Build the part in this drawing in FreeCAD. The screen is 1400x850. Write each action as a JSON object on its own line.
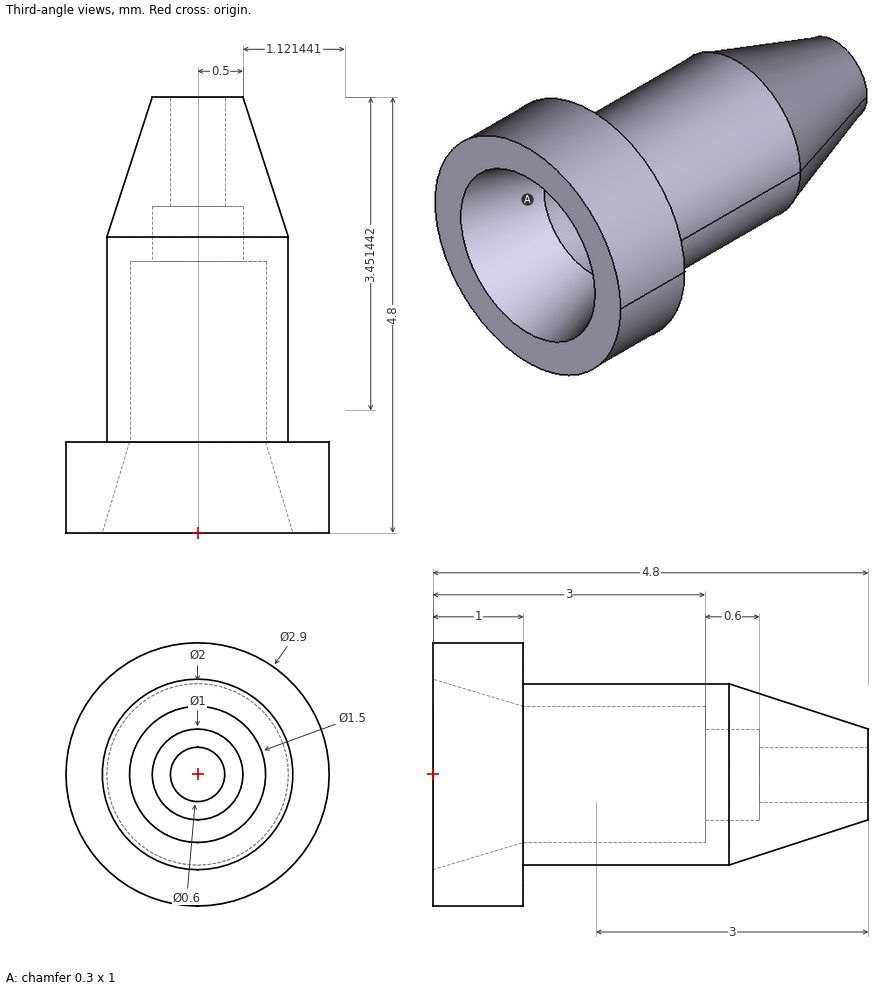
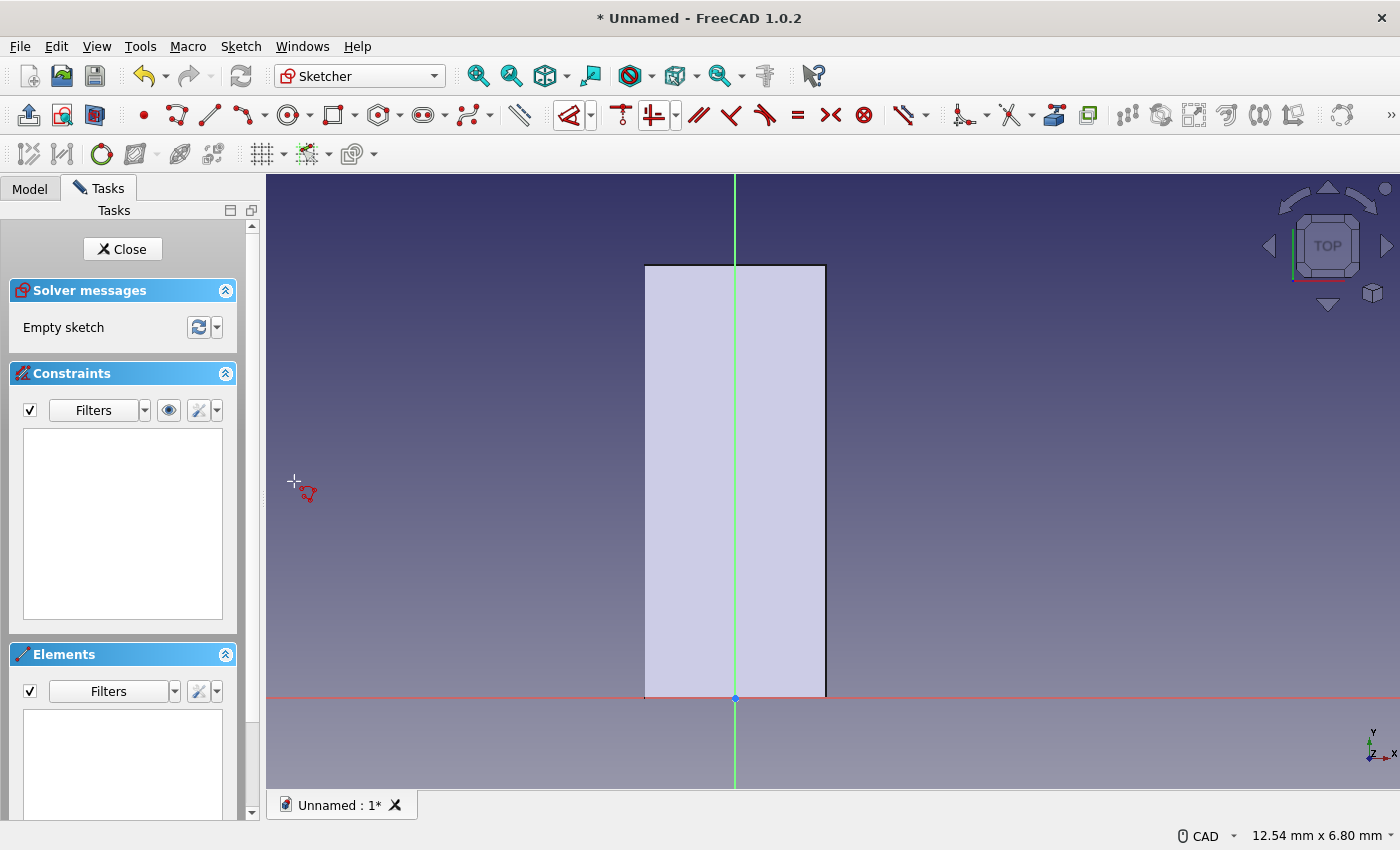
{"action": "left_click", "coordinate": [882, 577]}
{"action": "left_click", "coordinate": [882, 265]}
{"action": "left_click", "coordinate": [781, 265]}
{"action": "left_click", "coordinate": [882, 578]}
{"action": "key", "text": "Escape"}
{"action": "key", "text": "Escape"}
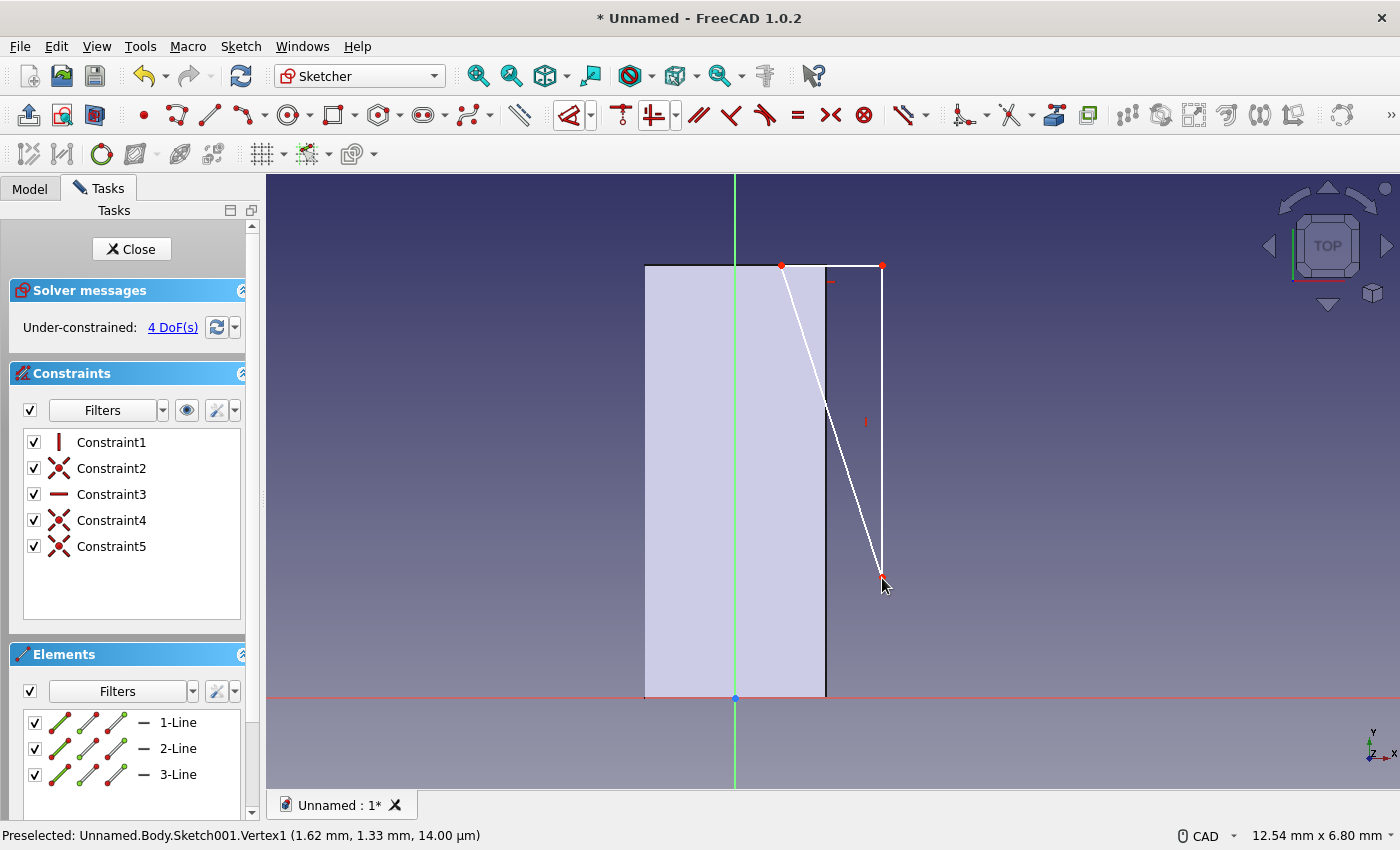
{"action": "left_click", "coordinate": [882, 266]}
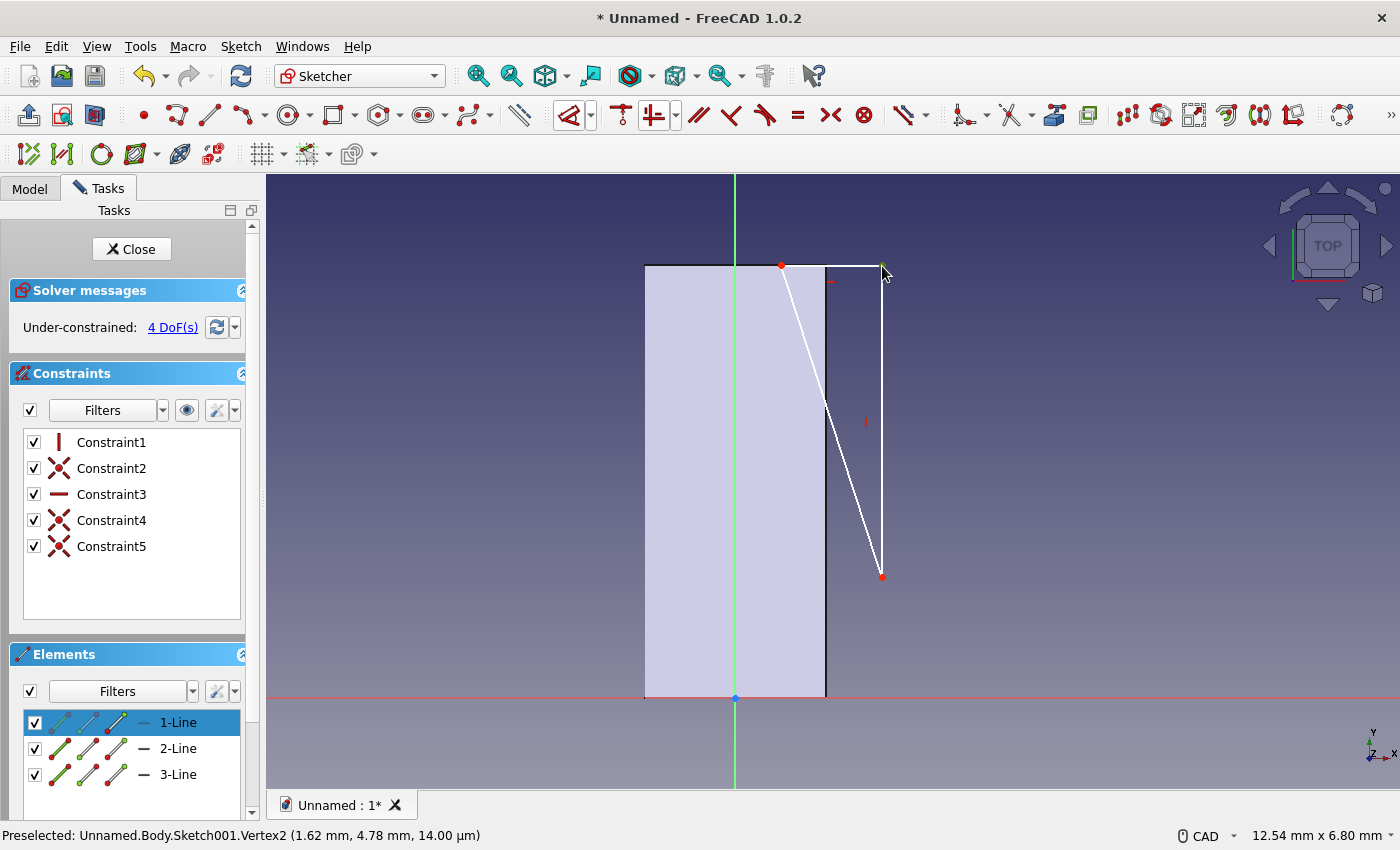
{"action": "key", "text": "i"}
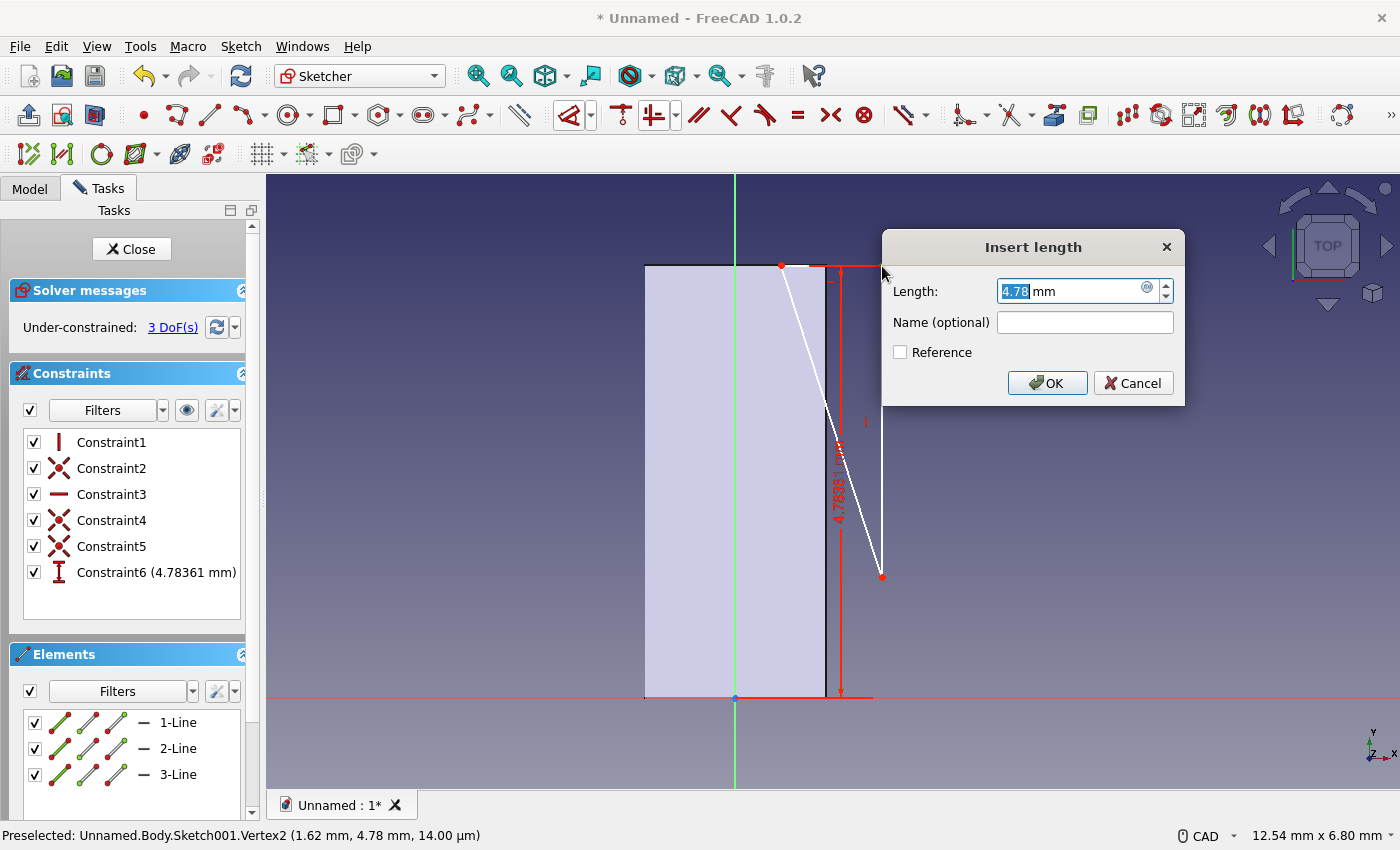
{"action": "type", "text": "4.8"}
{"action": "key", "text": "Return"}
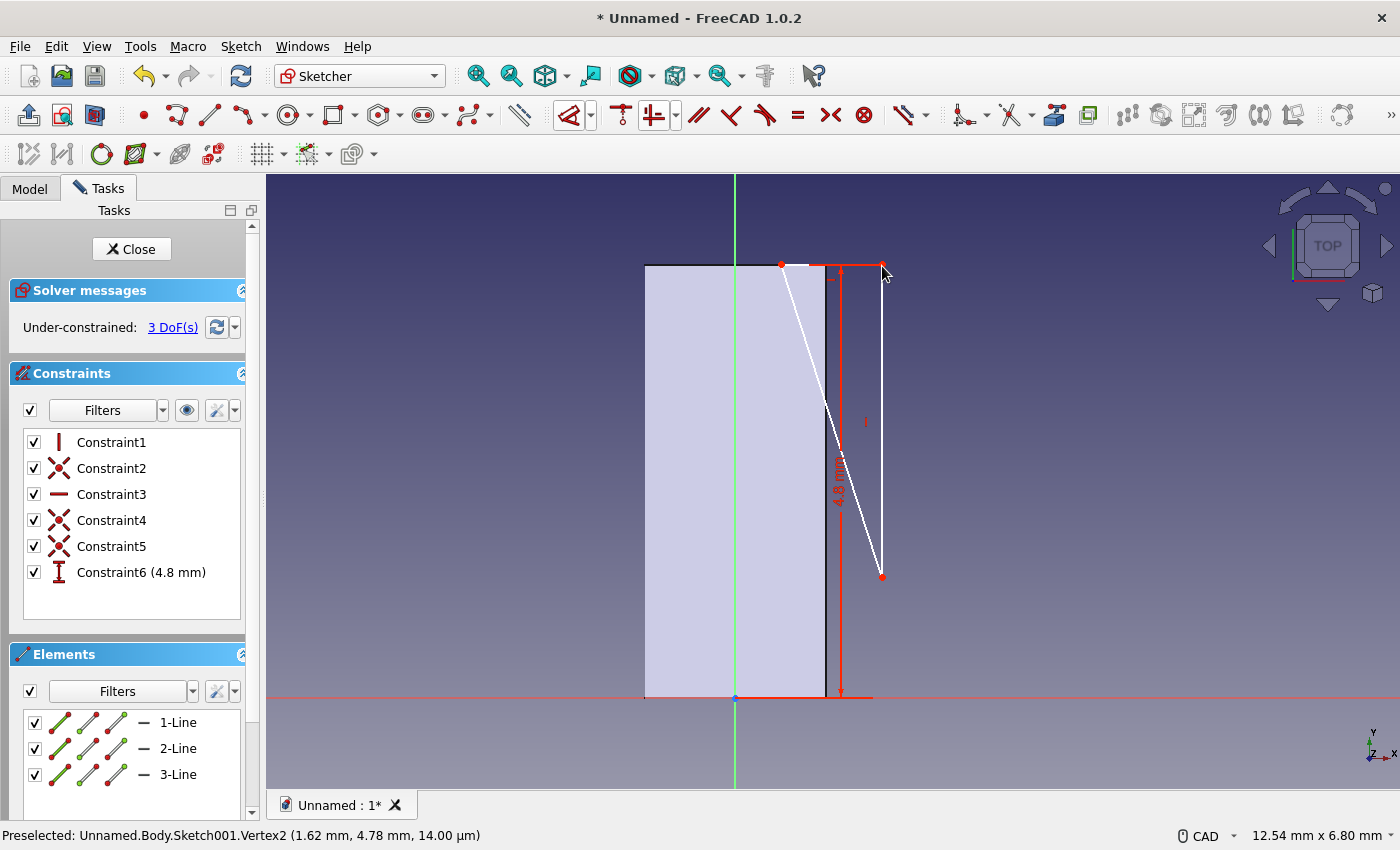
{"action": "left_click", "coordinate": [781, 265]}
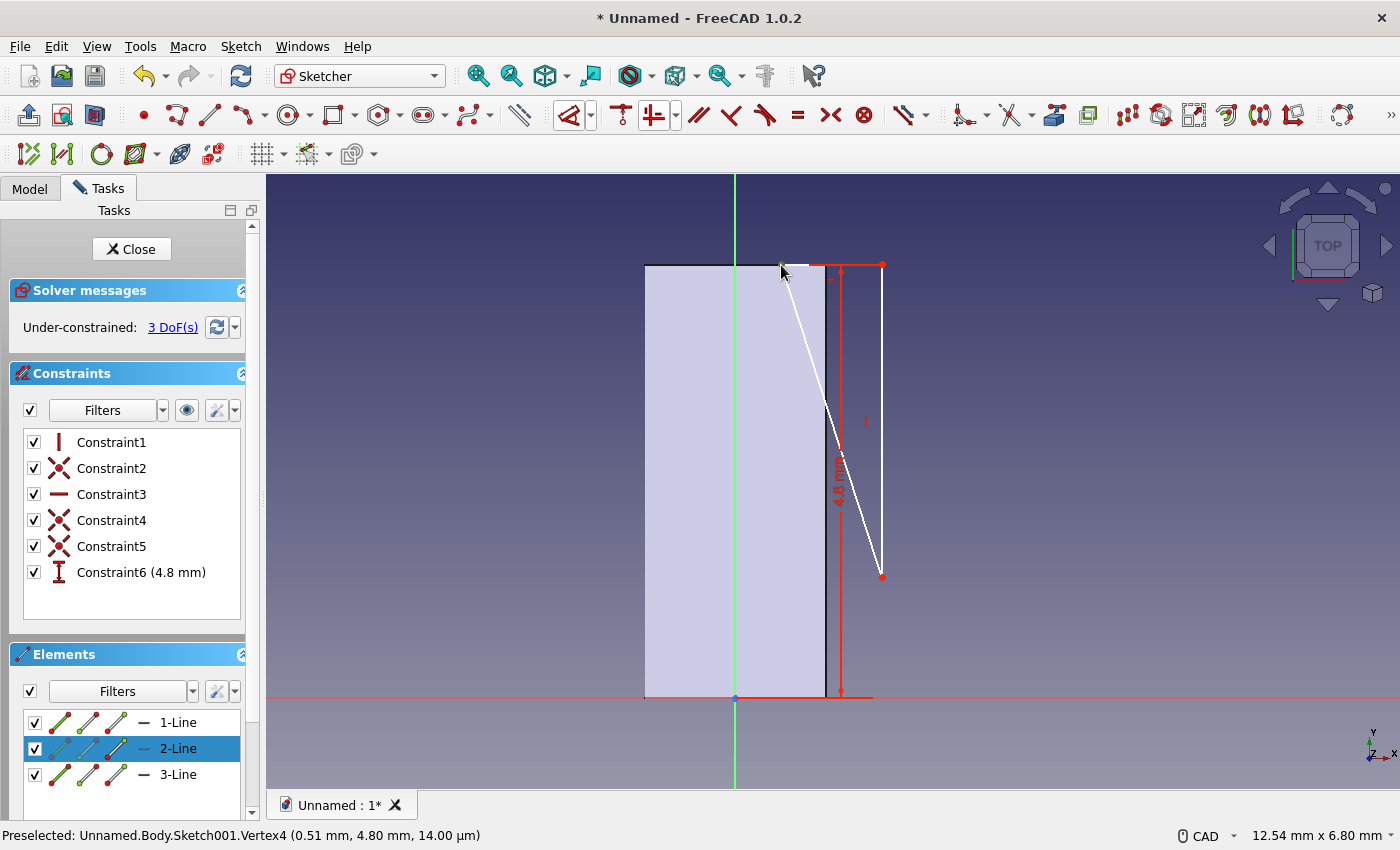
{"action": "key", "text": "l"}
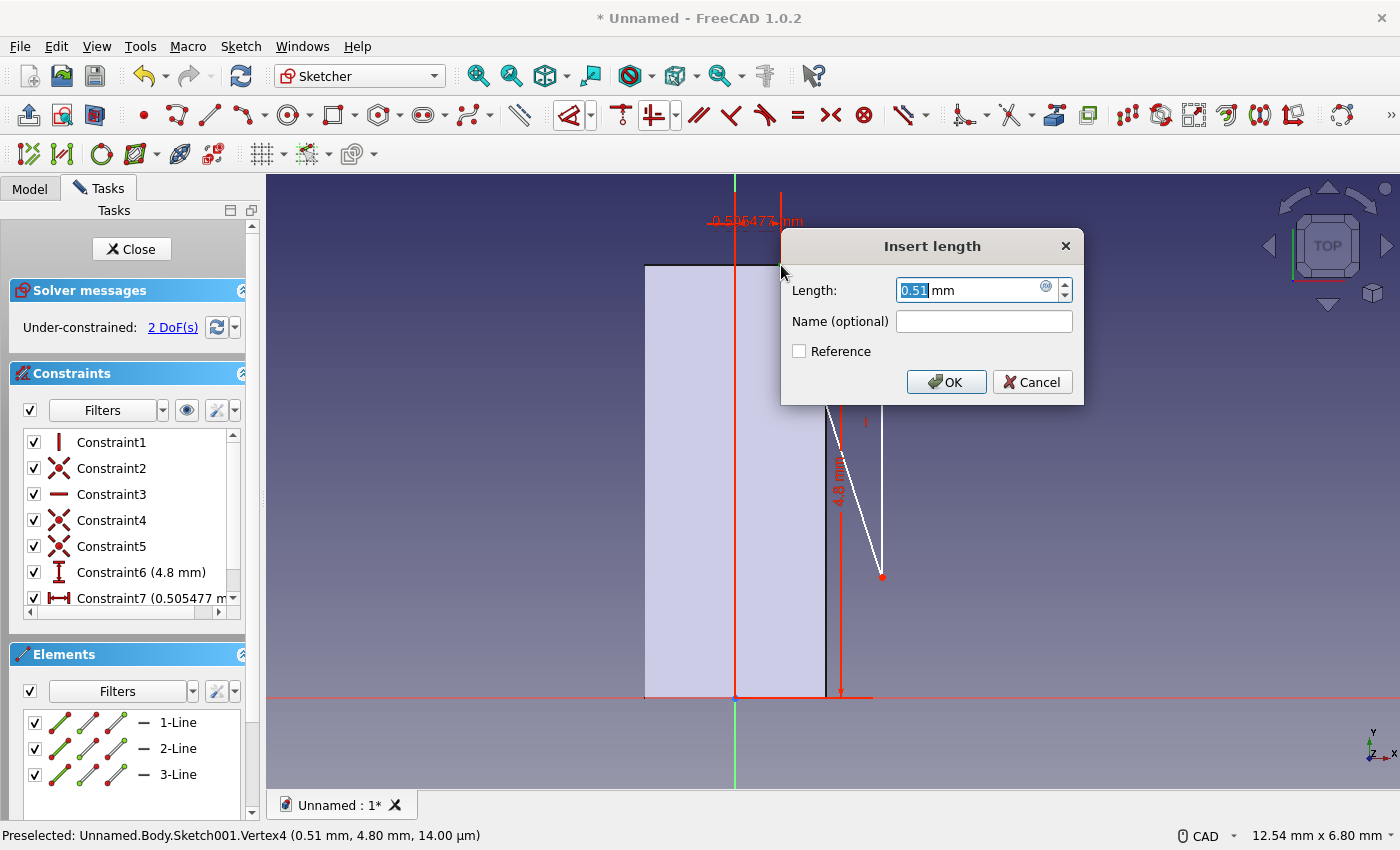
{"action": "type", "text": "0.5"}
{"action": "key", "text": "Return"}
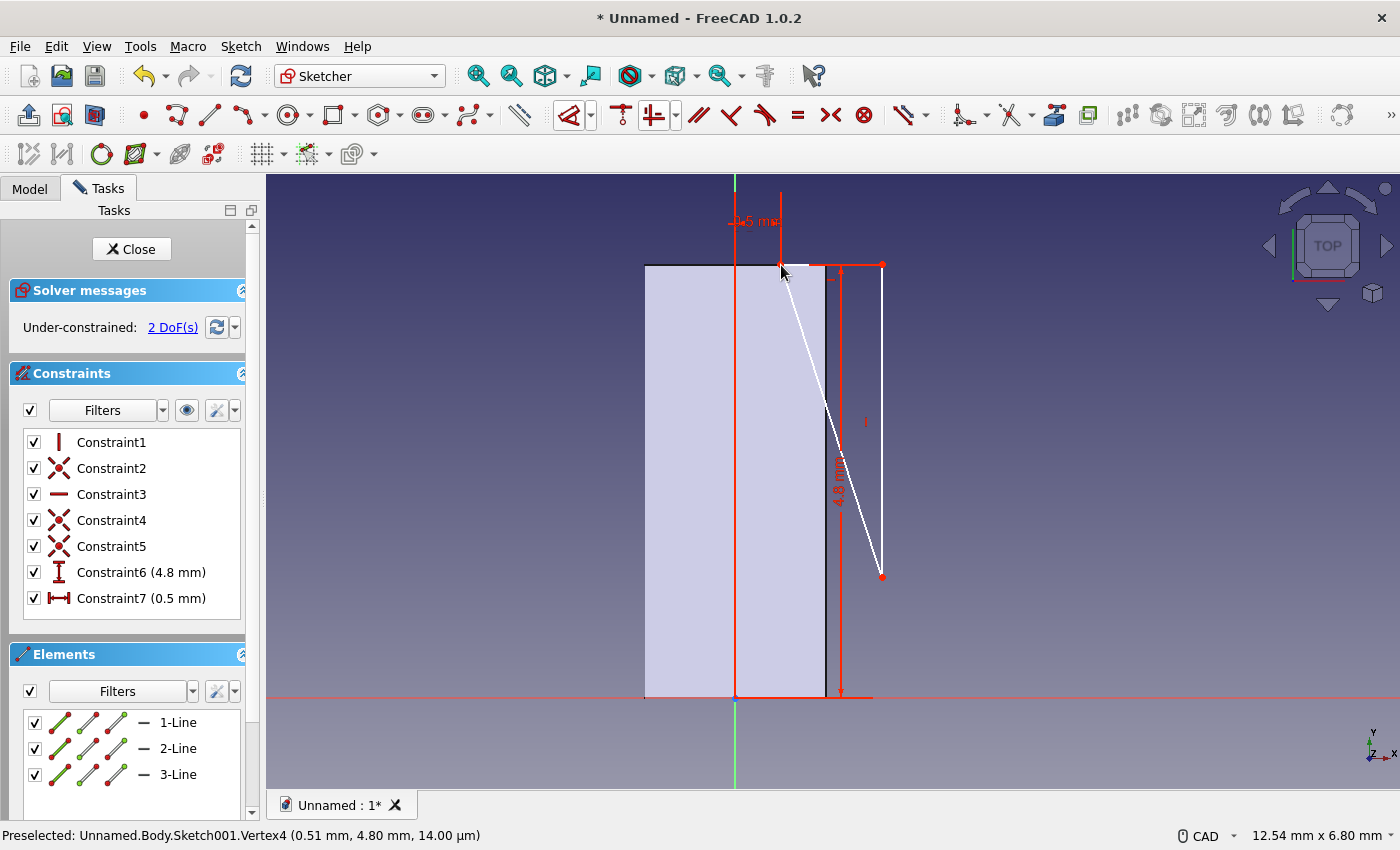
{"action": "left_click", "coordinate": [882, 484]}